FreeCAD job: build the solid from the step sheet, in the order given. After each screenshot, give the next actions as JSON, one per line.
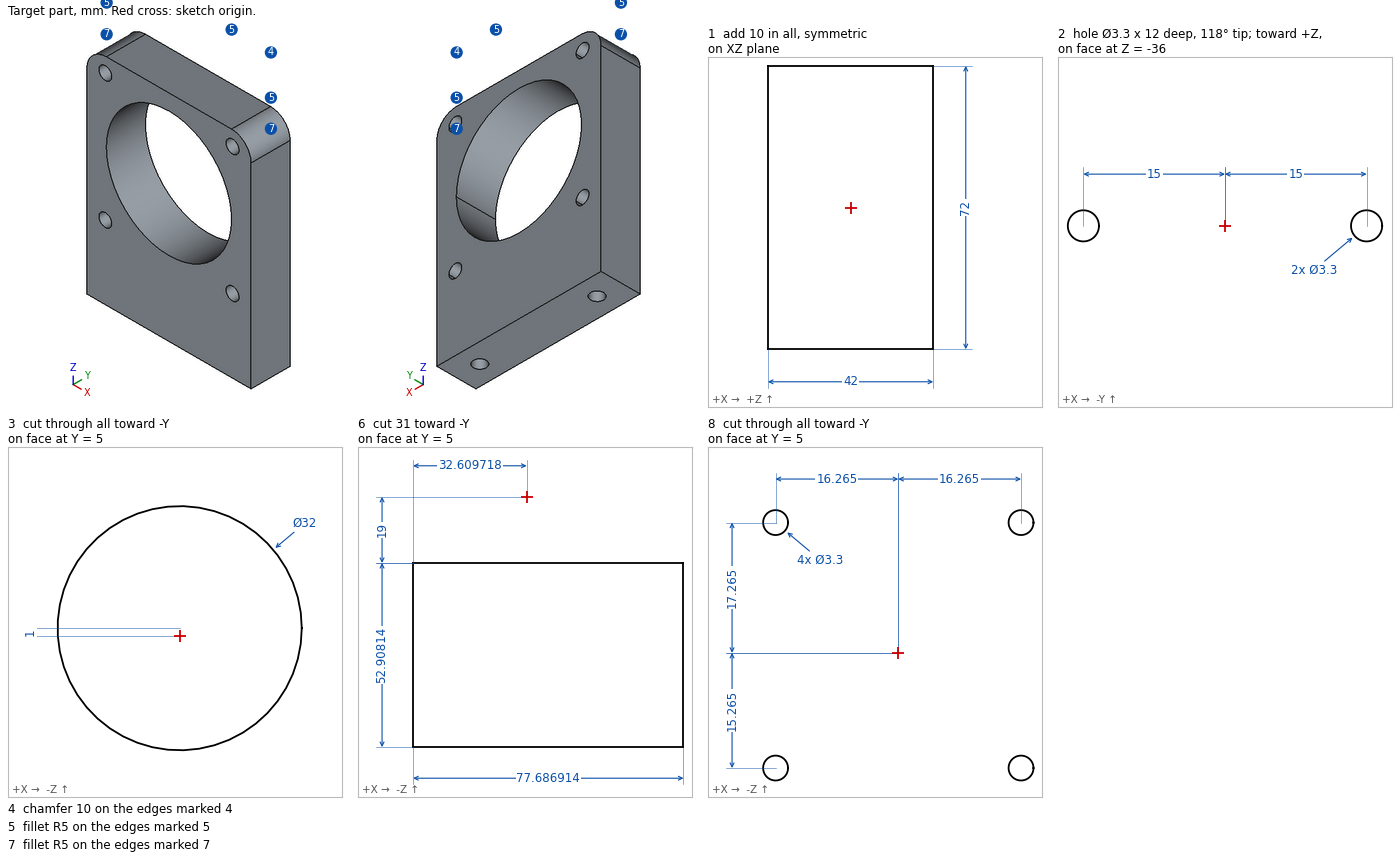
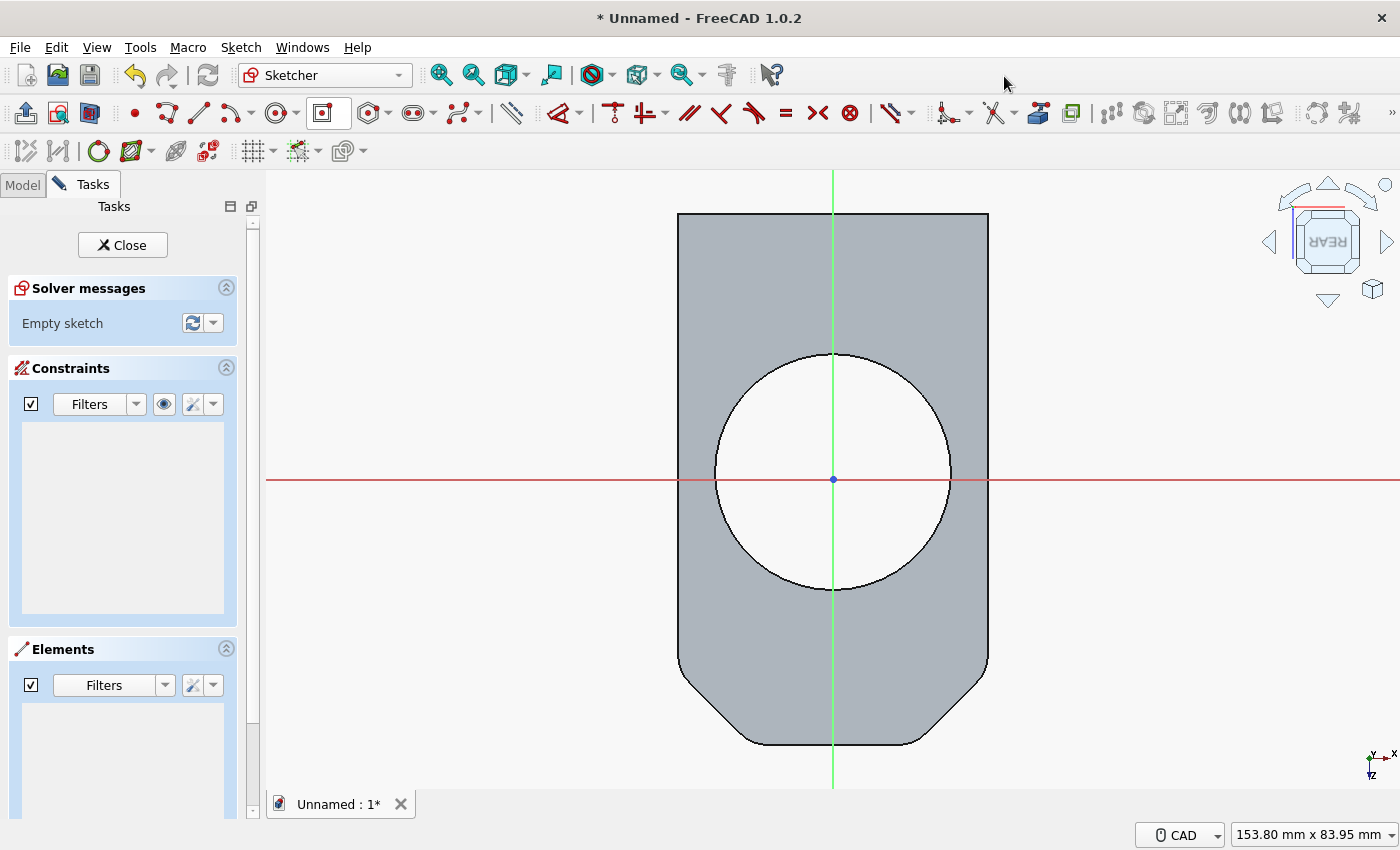
{"action": "scroll", "coordinate": [625, 198], "scroll_direction": "down", "scroll_amount": 3}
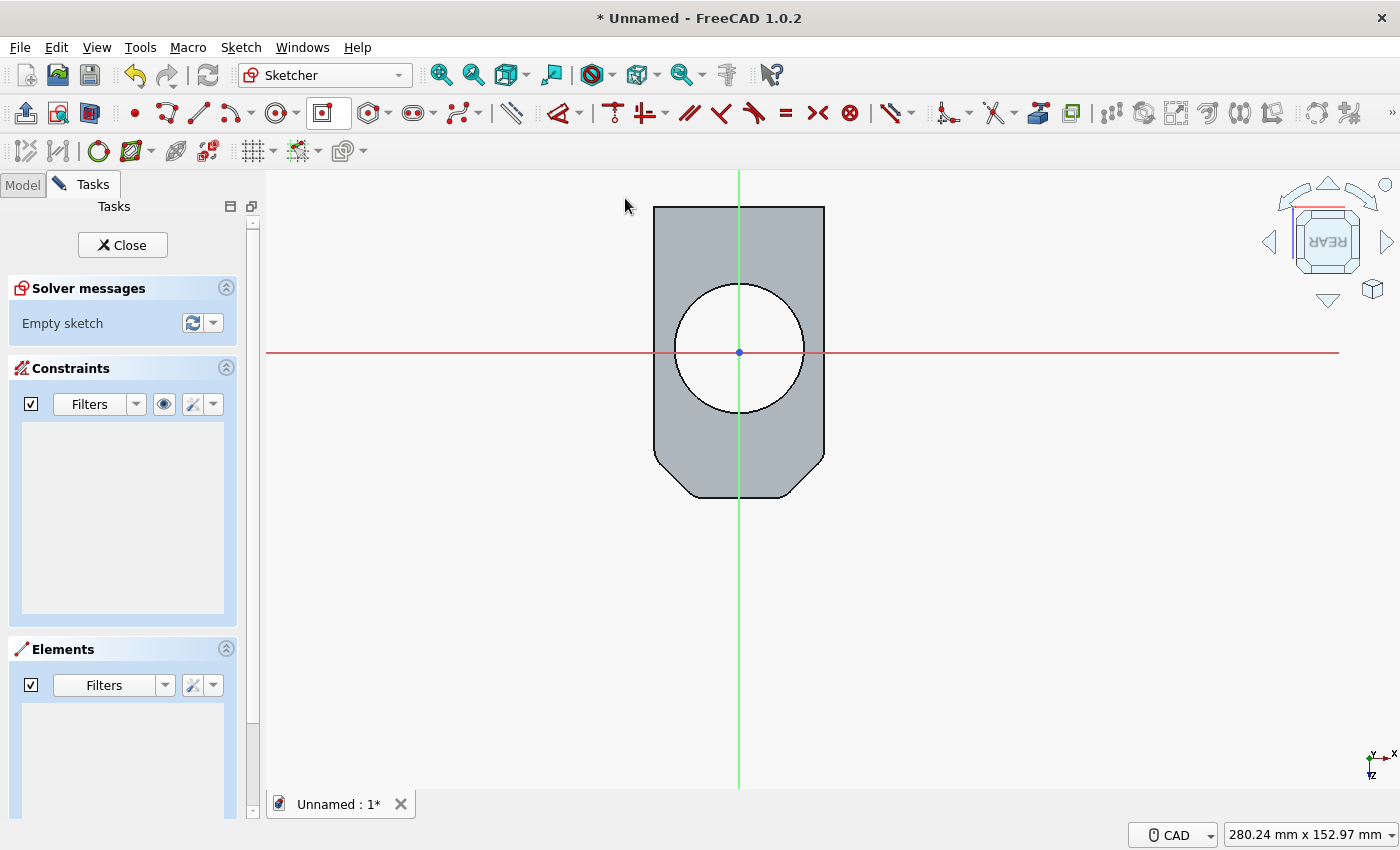
{"action": "scroll", "coordinate": [765, 536], "scroll_direction": "up", "scroll_amount": 2}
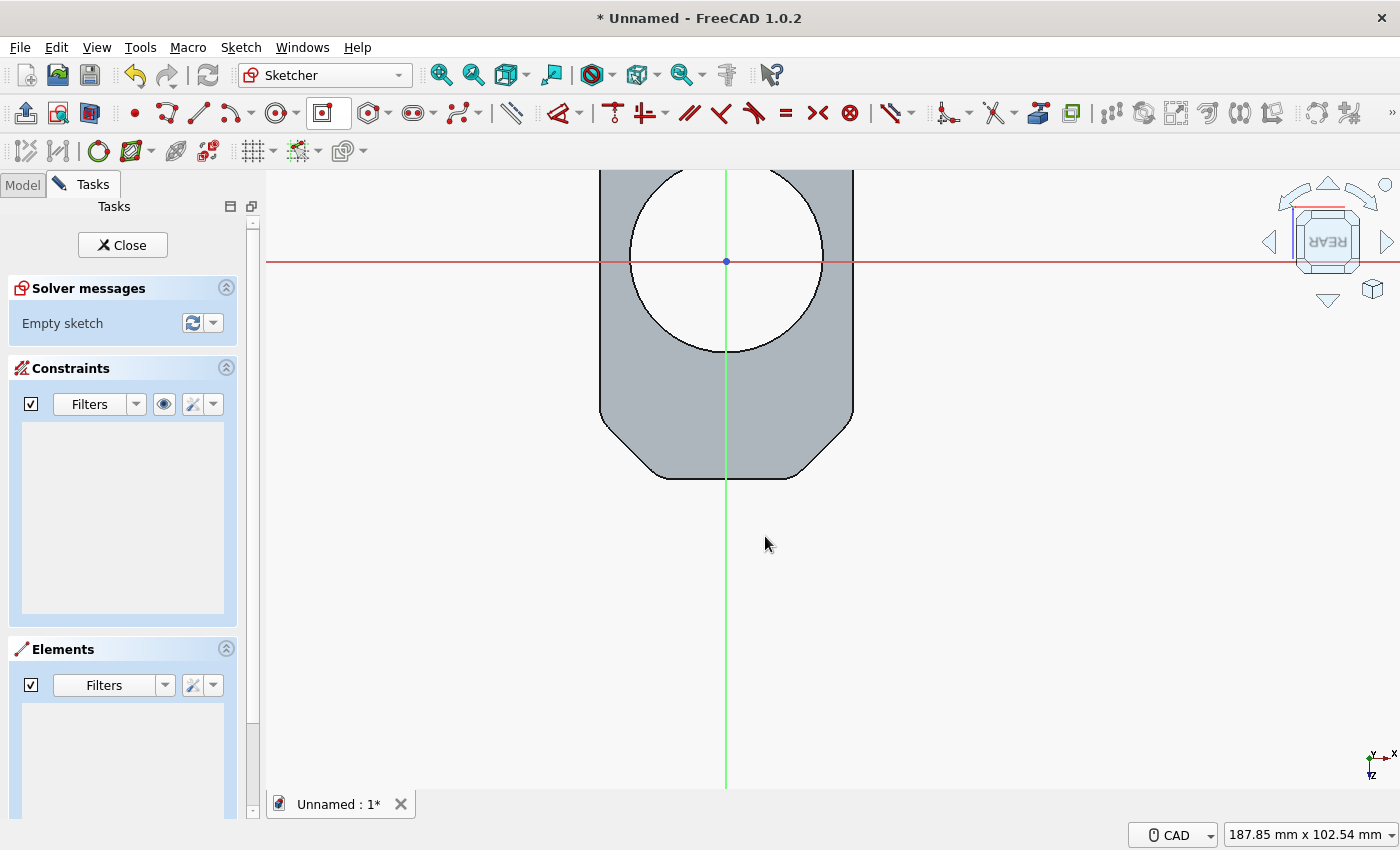
{"action": "left_click", "coordinate": [346, 114]}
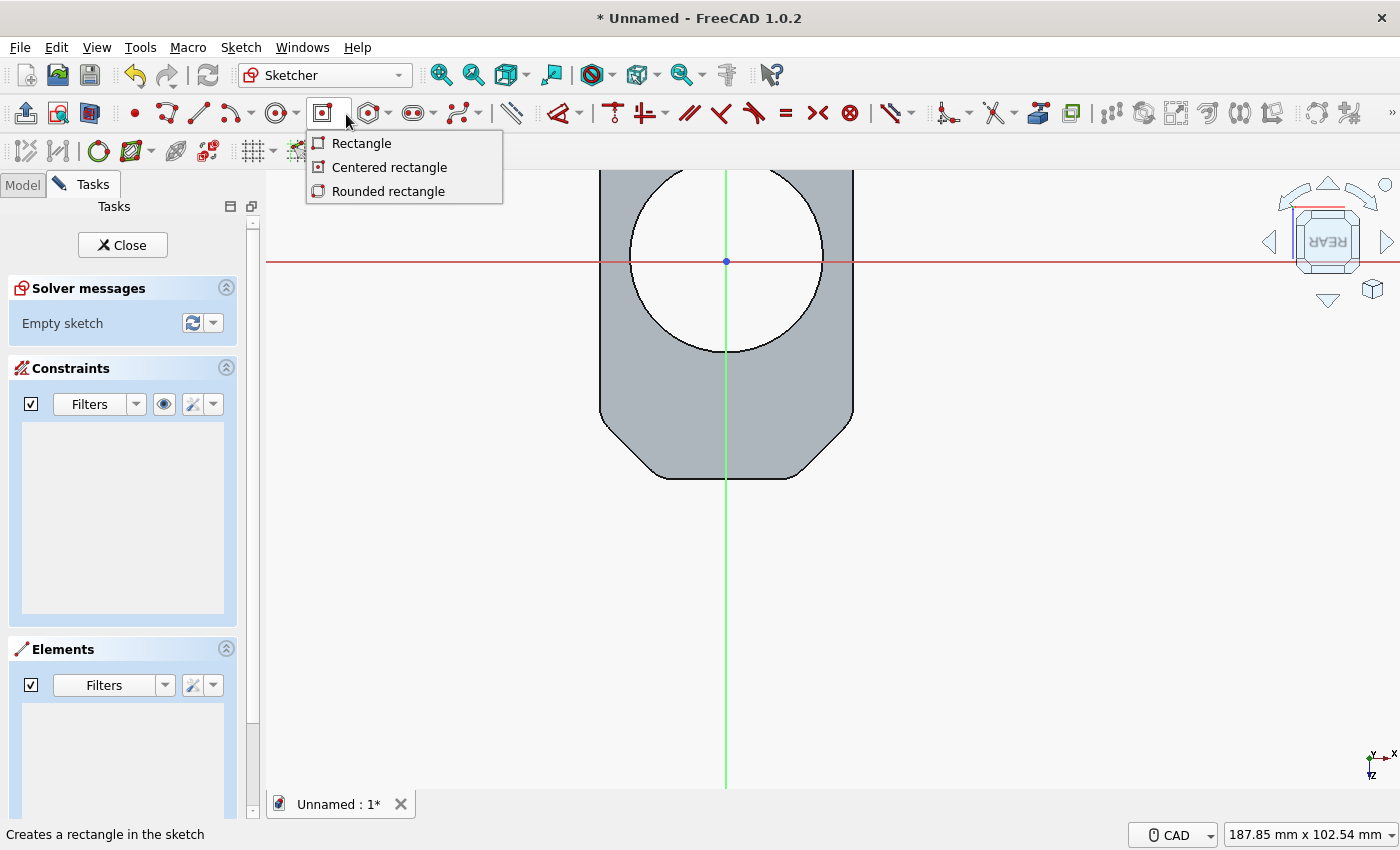
{"action": "left_click", "coordinate": [404, 143]}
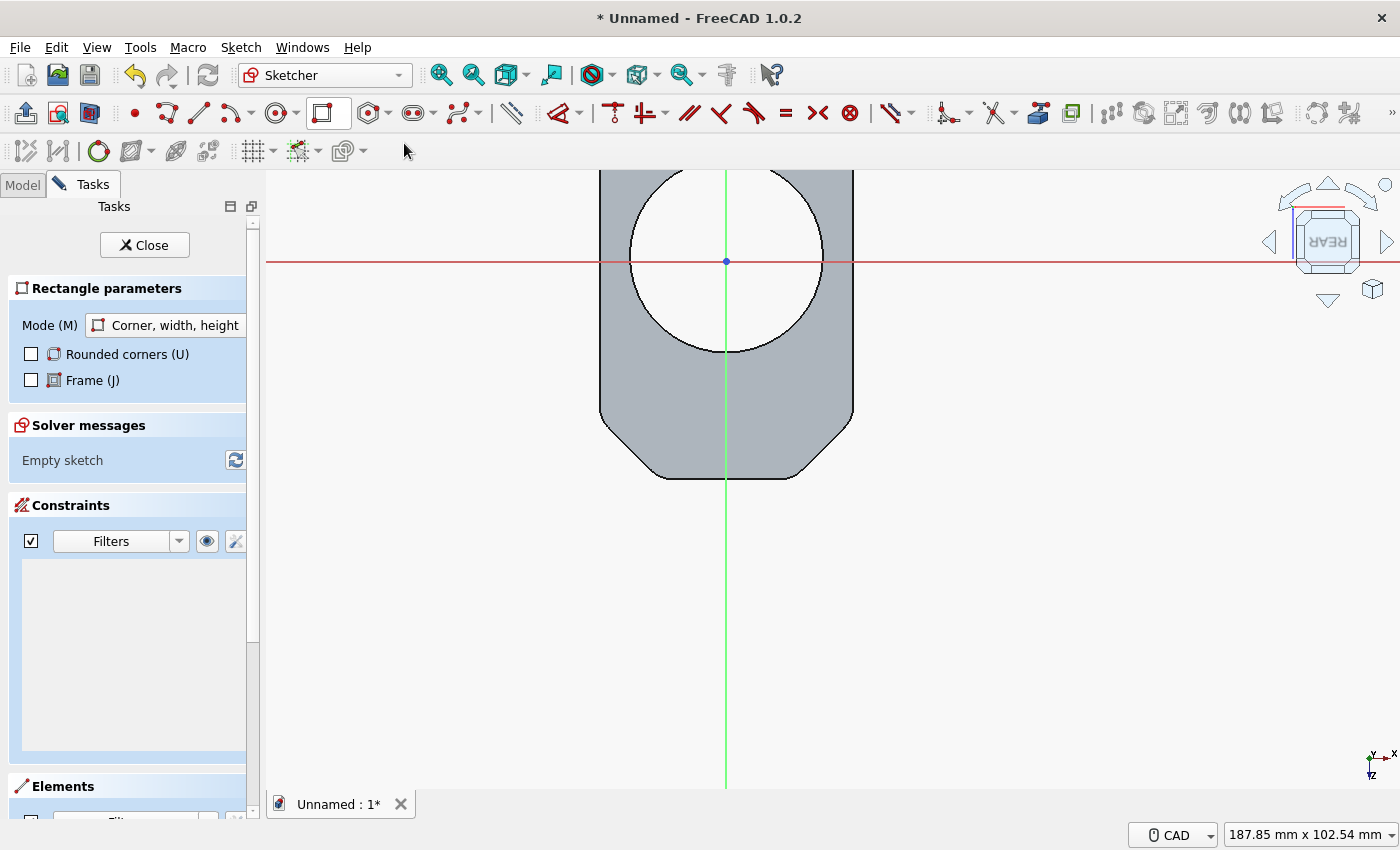
{"action": "left_click", "coordinate": [530, 377]}
{"action": "left_click", "coordinate": [999, 696]}
{"action": "key", "text": "Escape"}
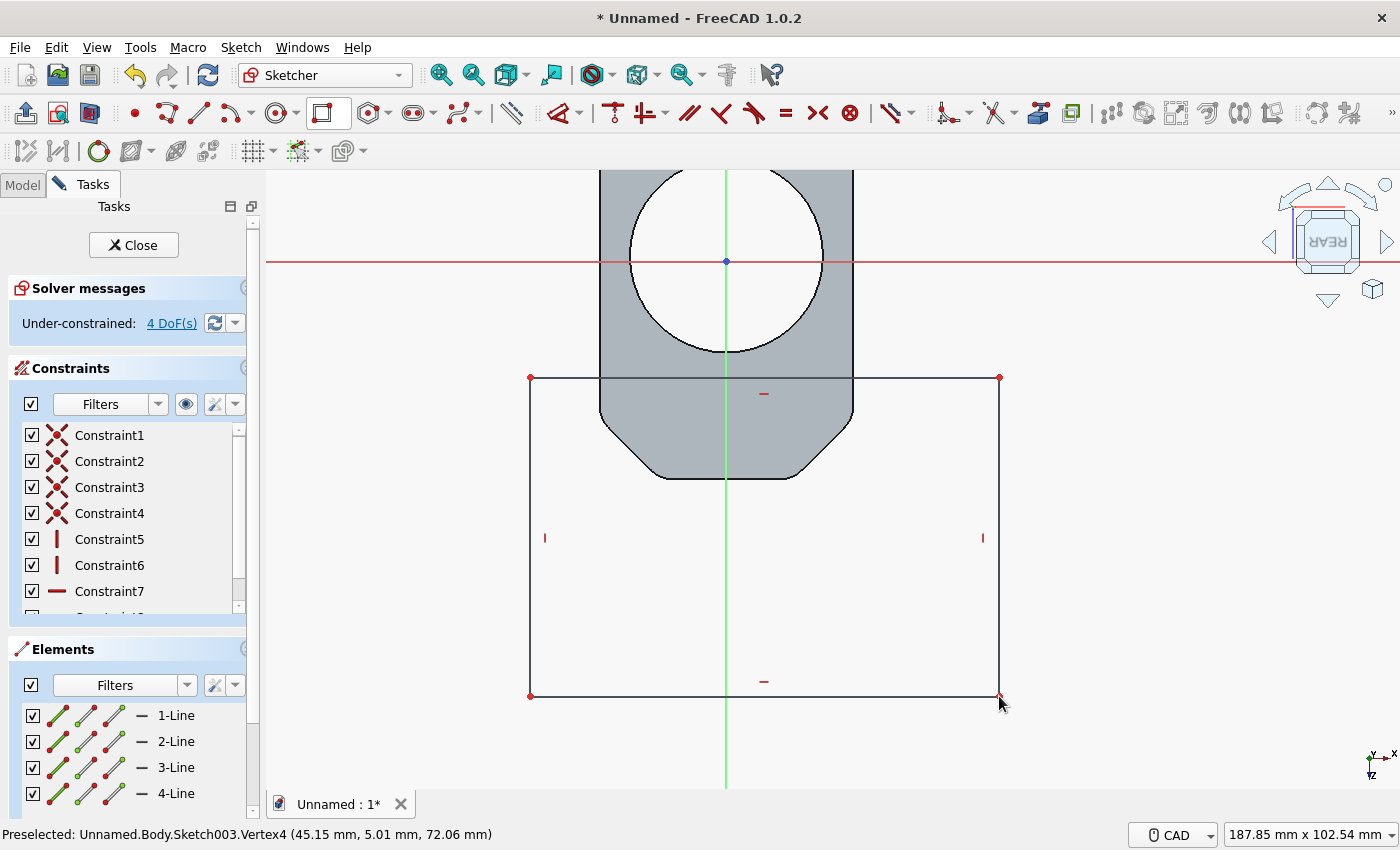
{"action": "left_click", "coordinate": [558, 114]}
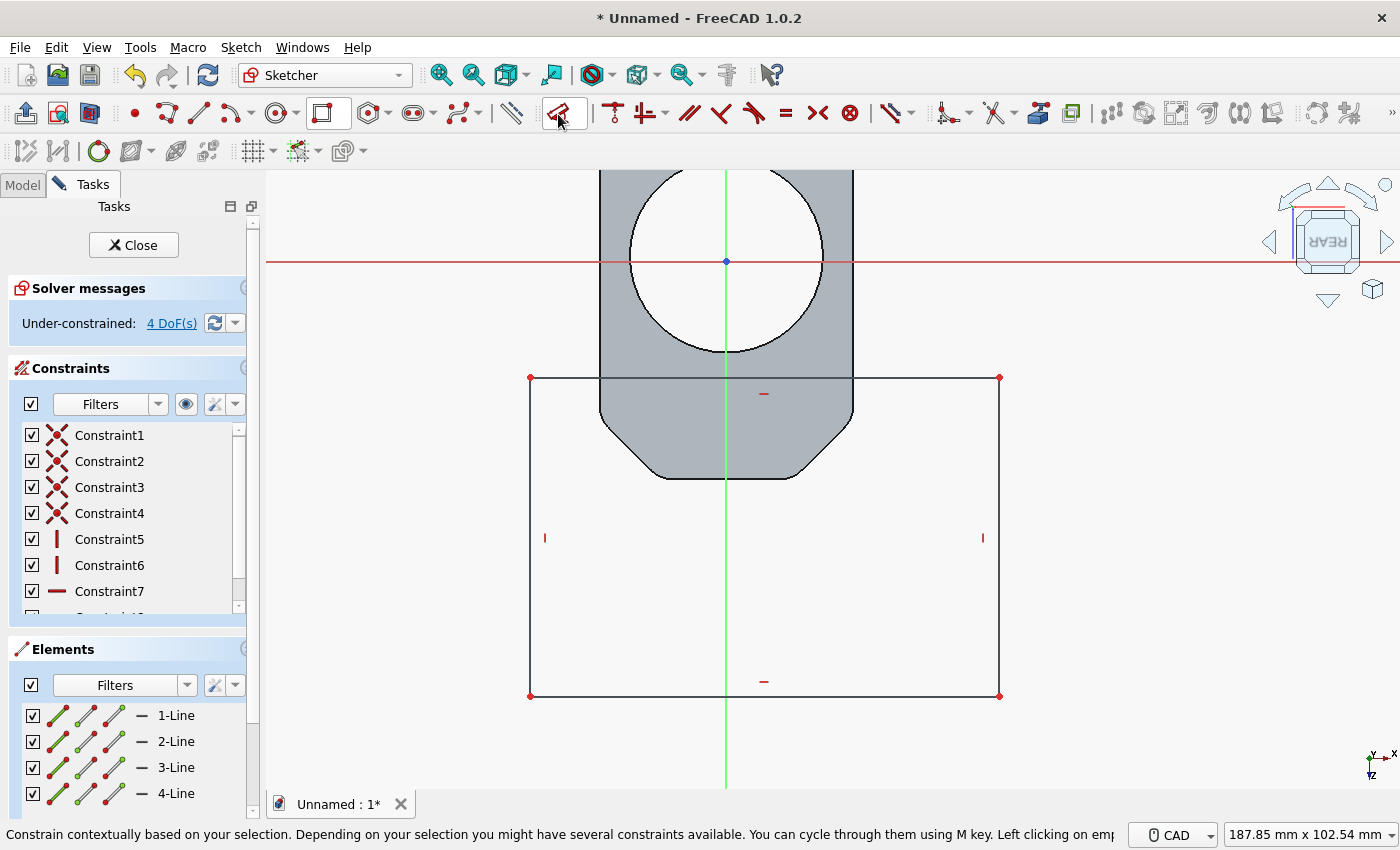
{"action": "left_click", "coordinate": [530, 378]}
{"action": "left_click", "coordinate": [496, 320]}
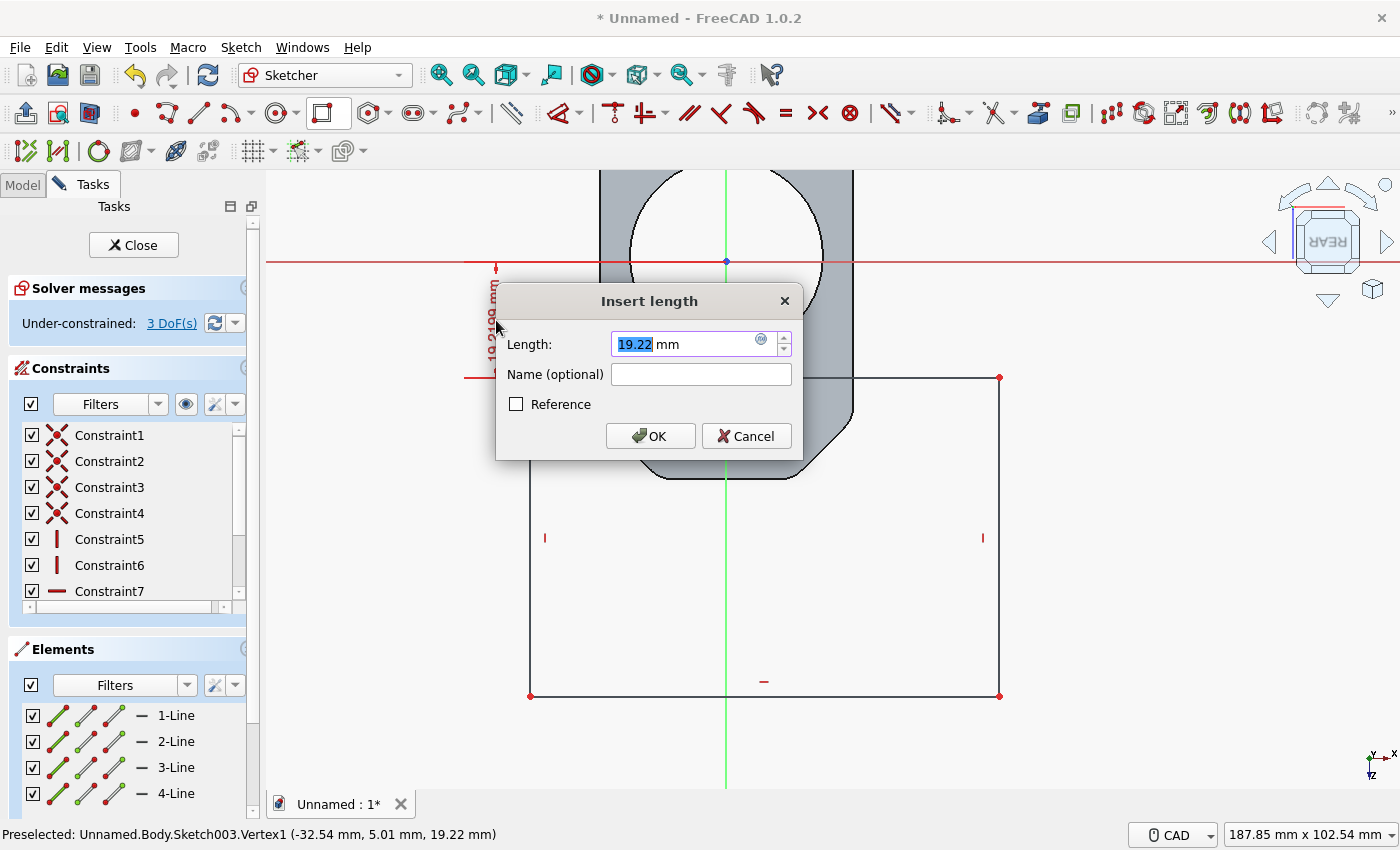
{"action": "type", "text": "19"}
{"action": "key", "text": "Return"}